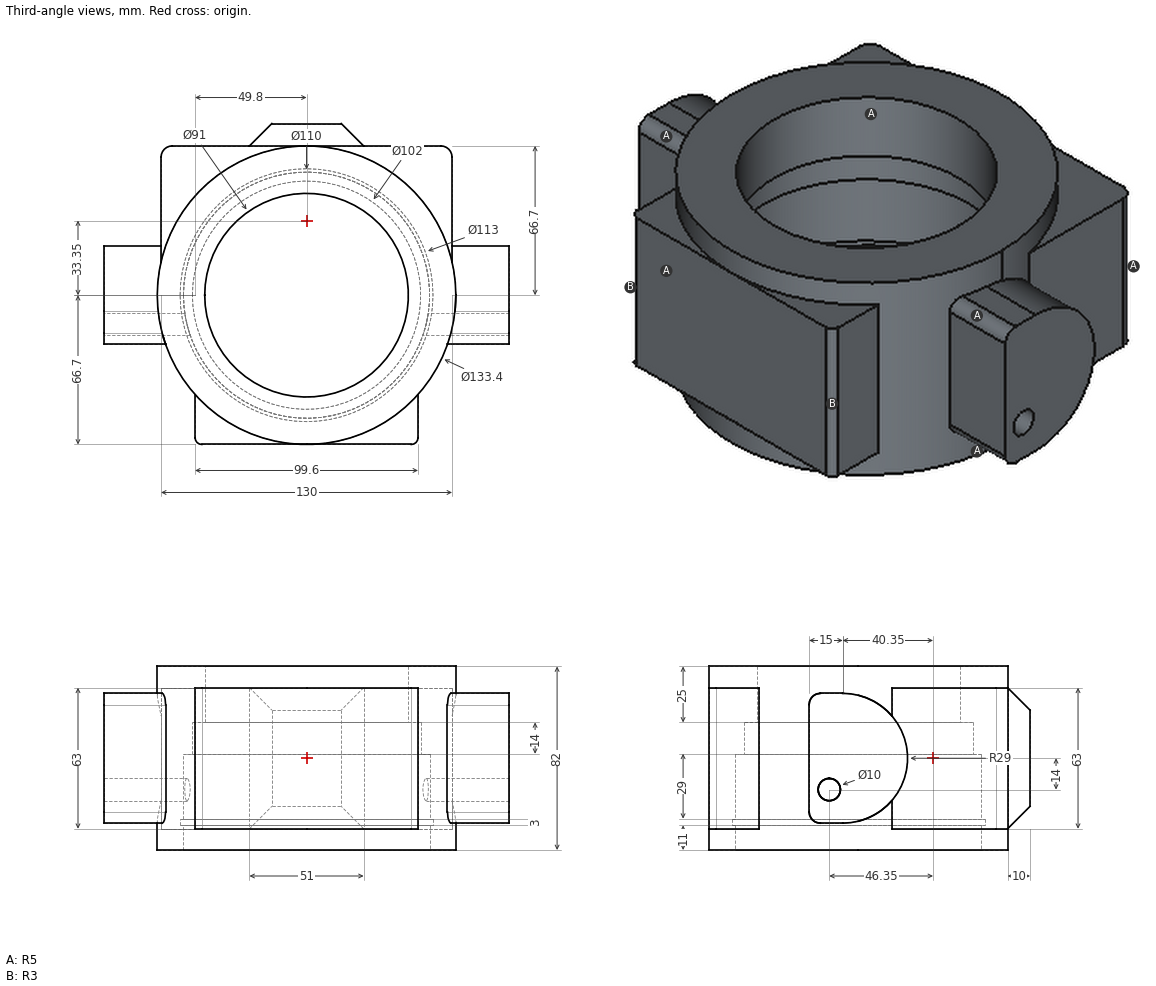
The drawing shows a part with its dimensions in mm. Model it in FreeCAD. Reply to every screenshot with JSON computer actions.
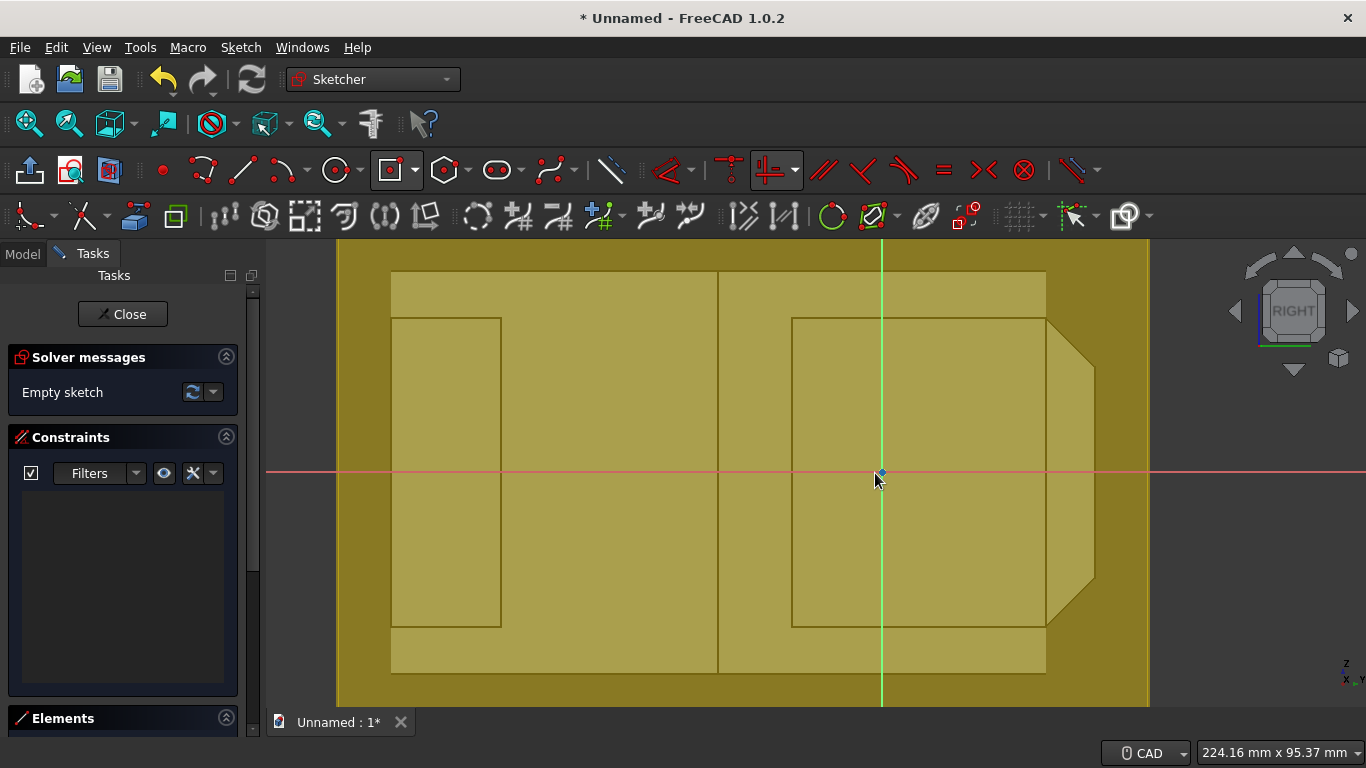
{"action": "key", "text": "g m"}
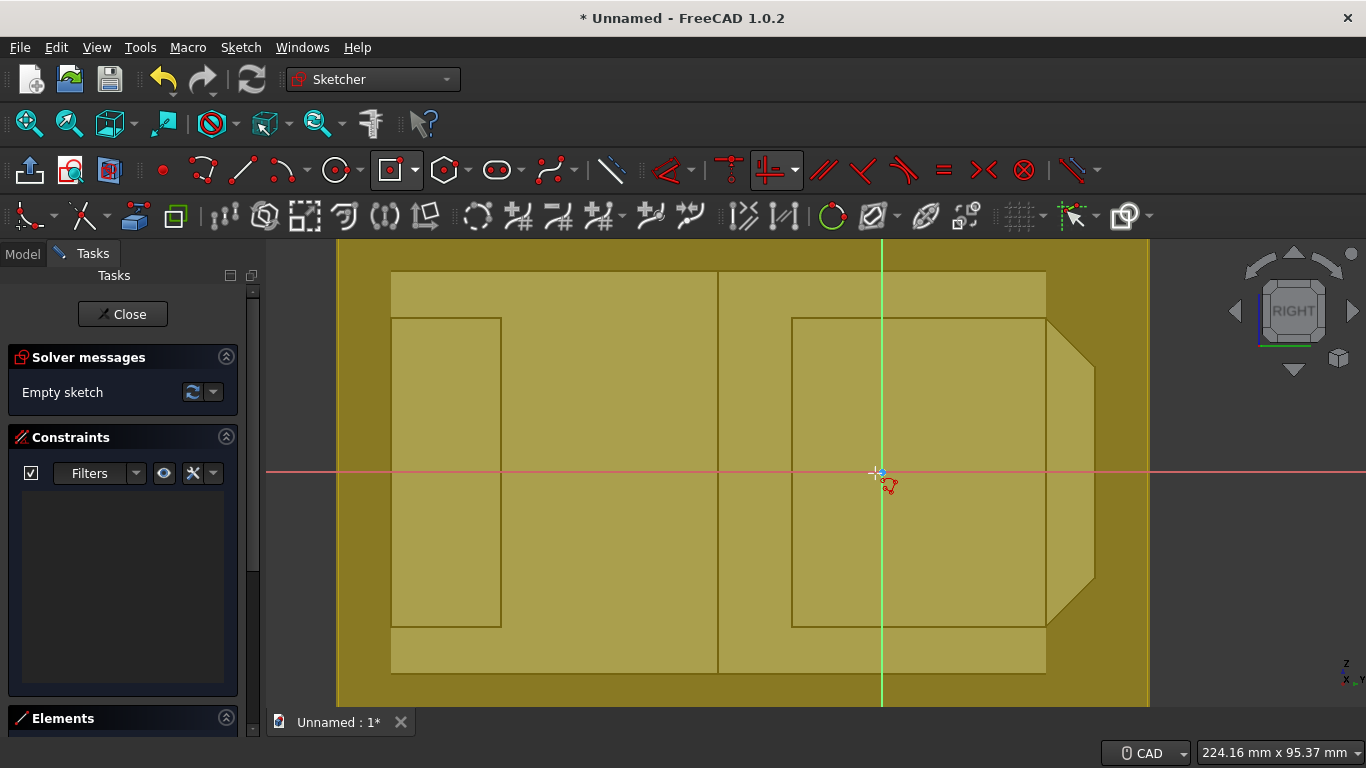
{"action": "left_click", "coordinate": [684, 330]}
{"action": "left_click", "coordinate": [611, 330]}
{"action": "left_click", "coordinate": [611, 615]}
{"action": "left_click", "coordinate": [684, 615]}
{"action": "right_click", "coordinate": [684, 615]}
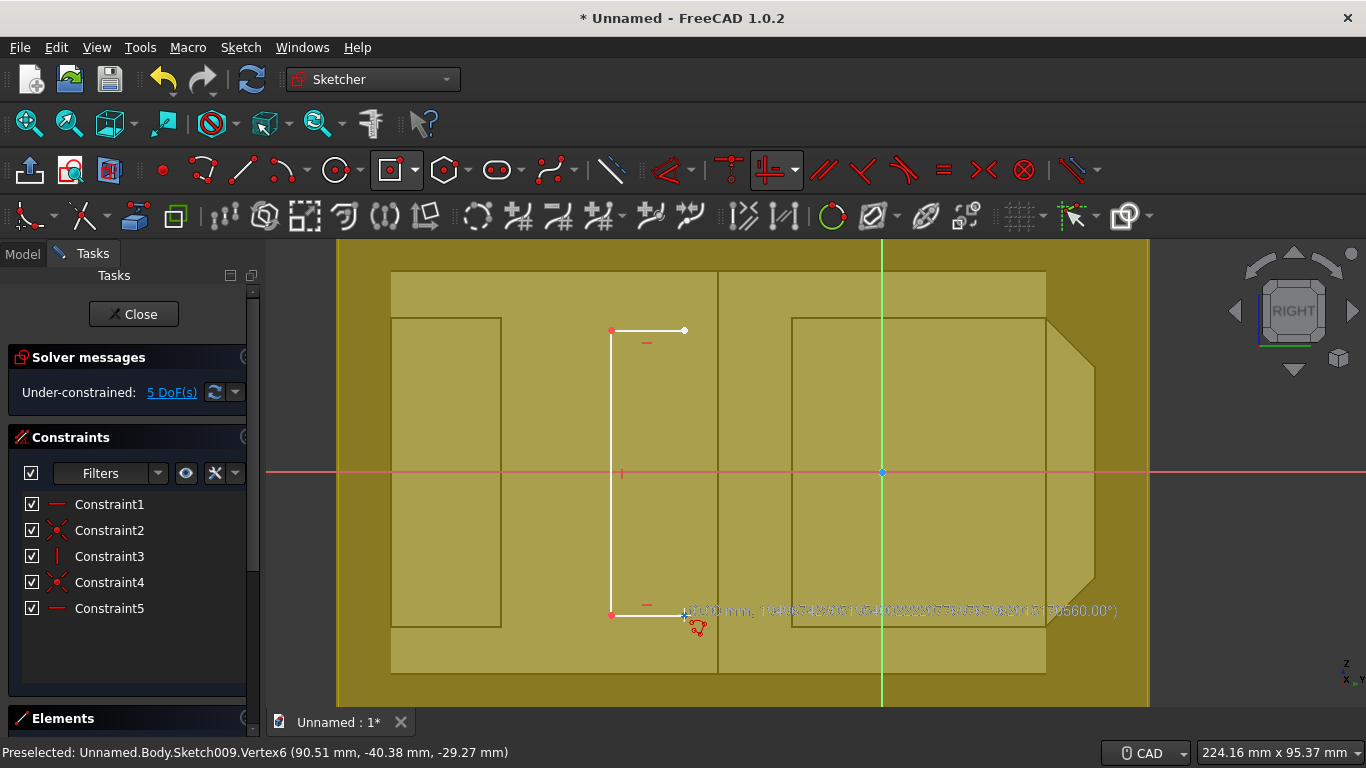
{"action": "key", "text": "g 3 a"}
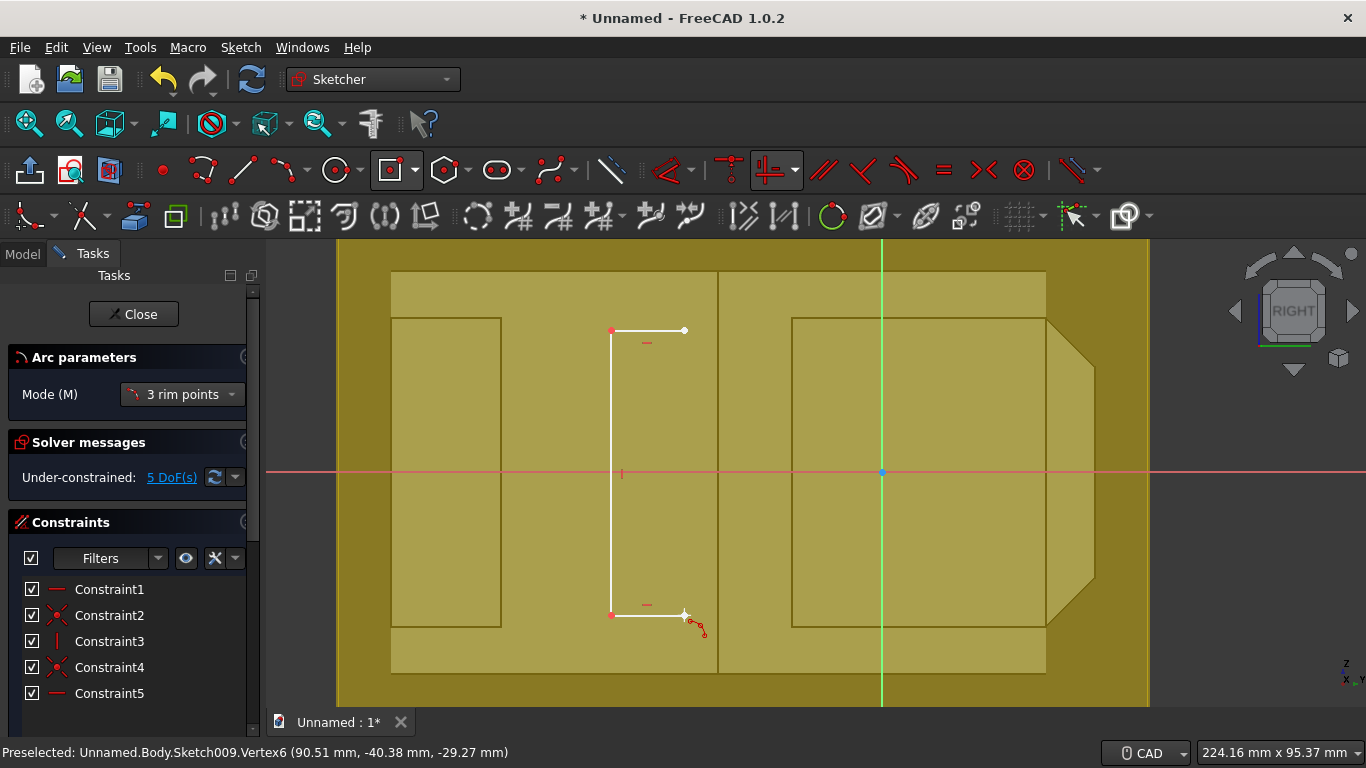
{"action": "left_click", "coordinate": [684, 616]}
{"action": "left_click", "coordinate": [684, 331]}
{"action": "left_click", "coordinate": [819, 516]}
{"action": "key", "text": "Escape"}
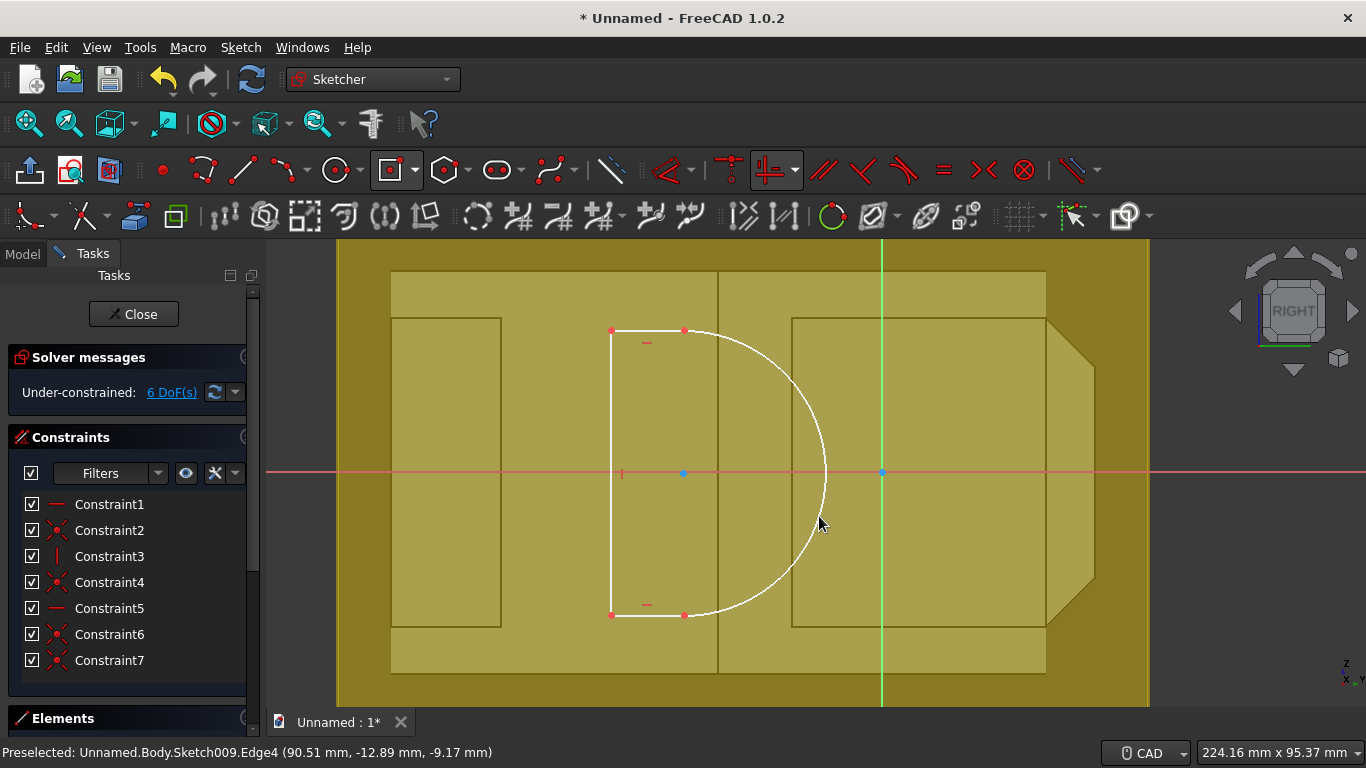
{"action": "left_click", "coordinate": [662, 331]}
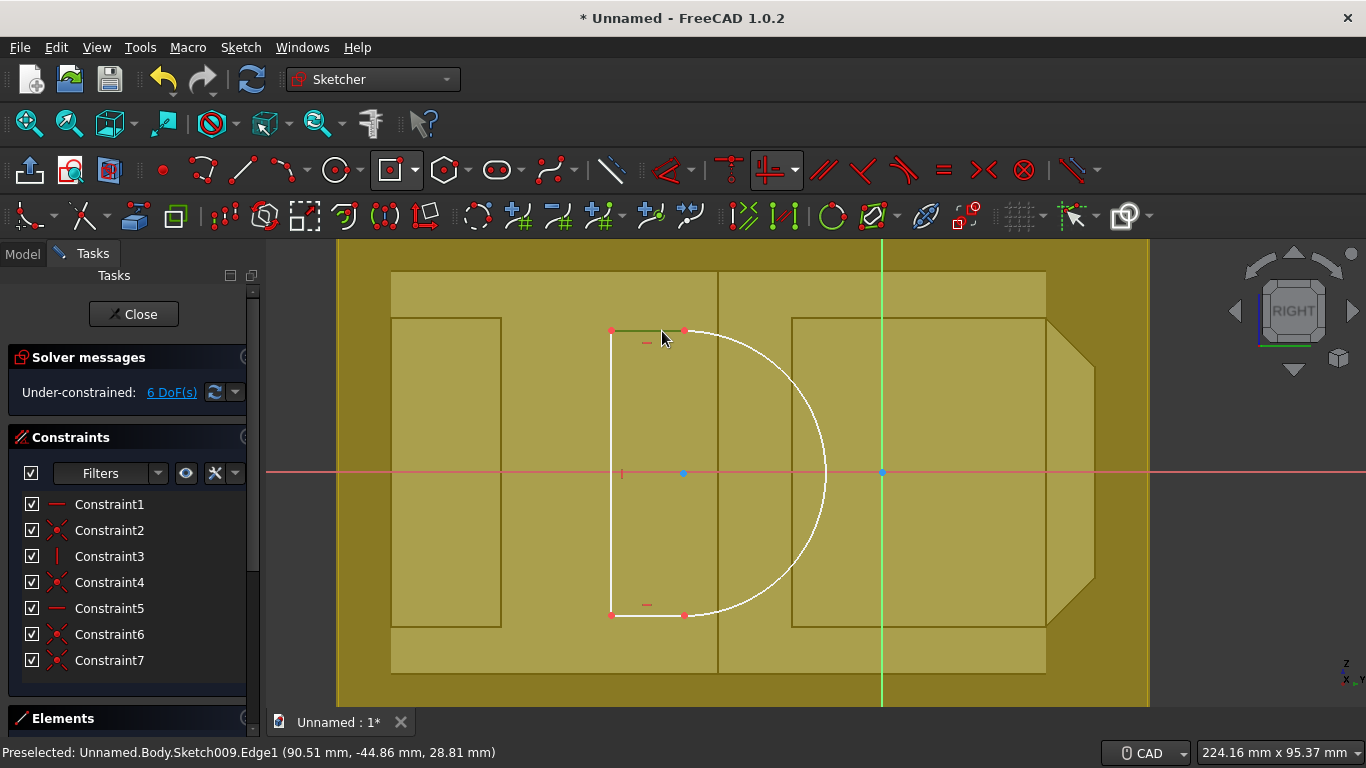
{"action": "left_click", "coordinate": [799, 557]}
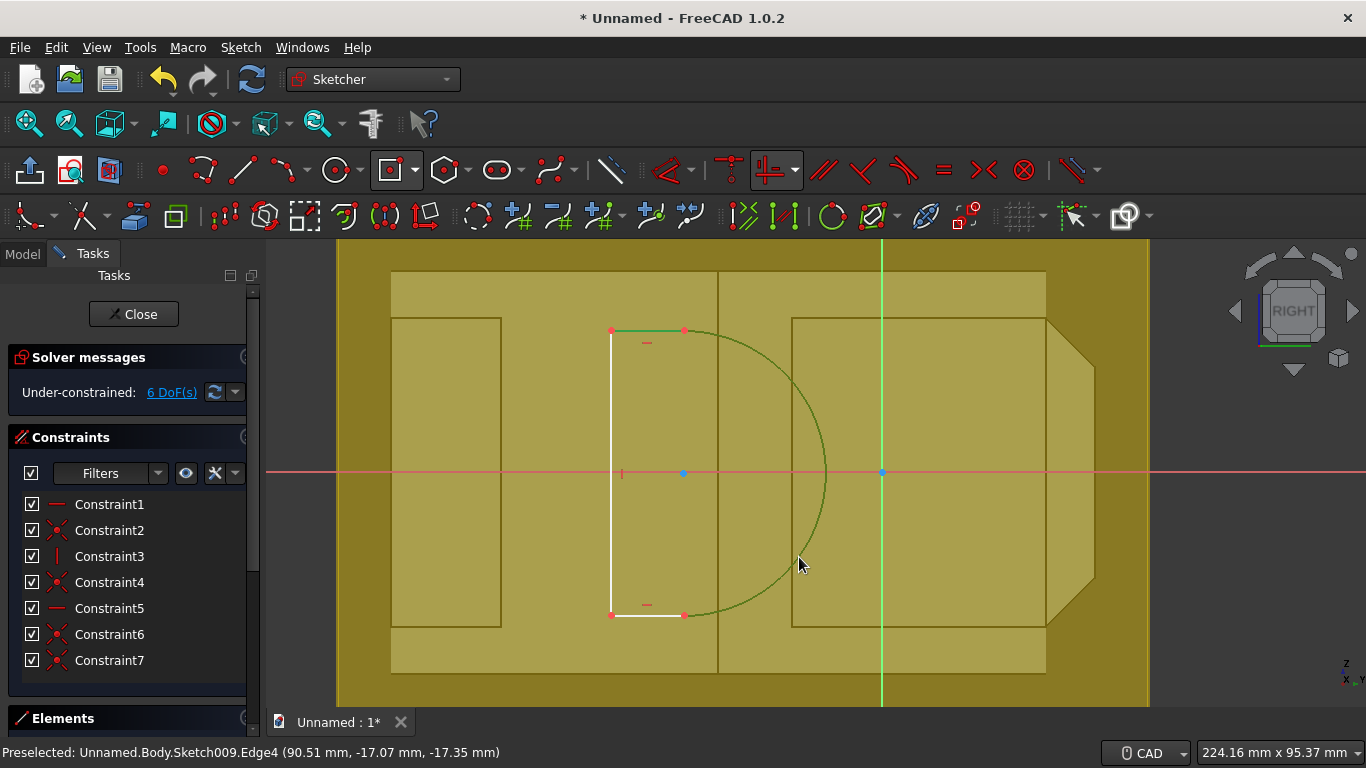
{"action": "key", "text": "t"}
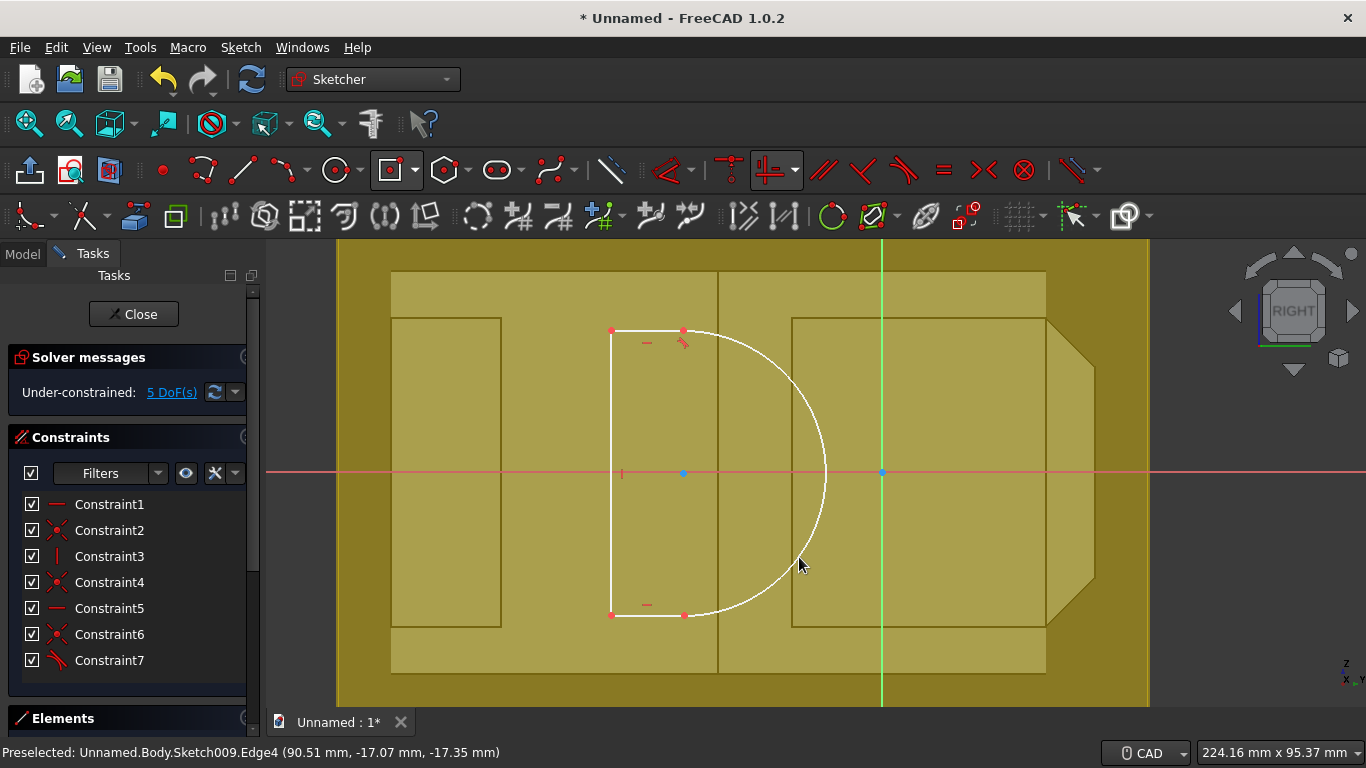
{"action": "left_click", "coordinate": [633, 616]}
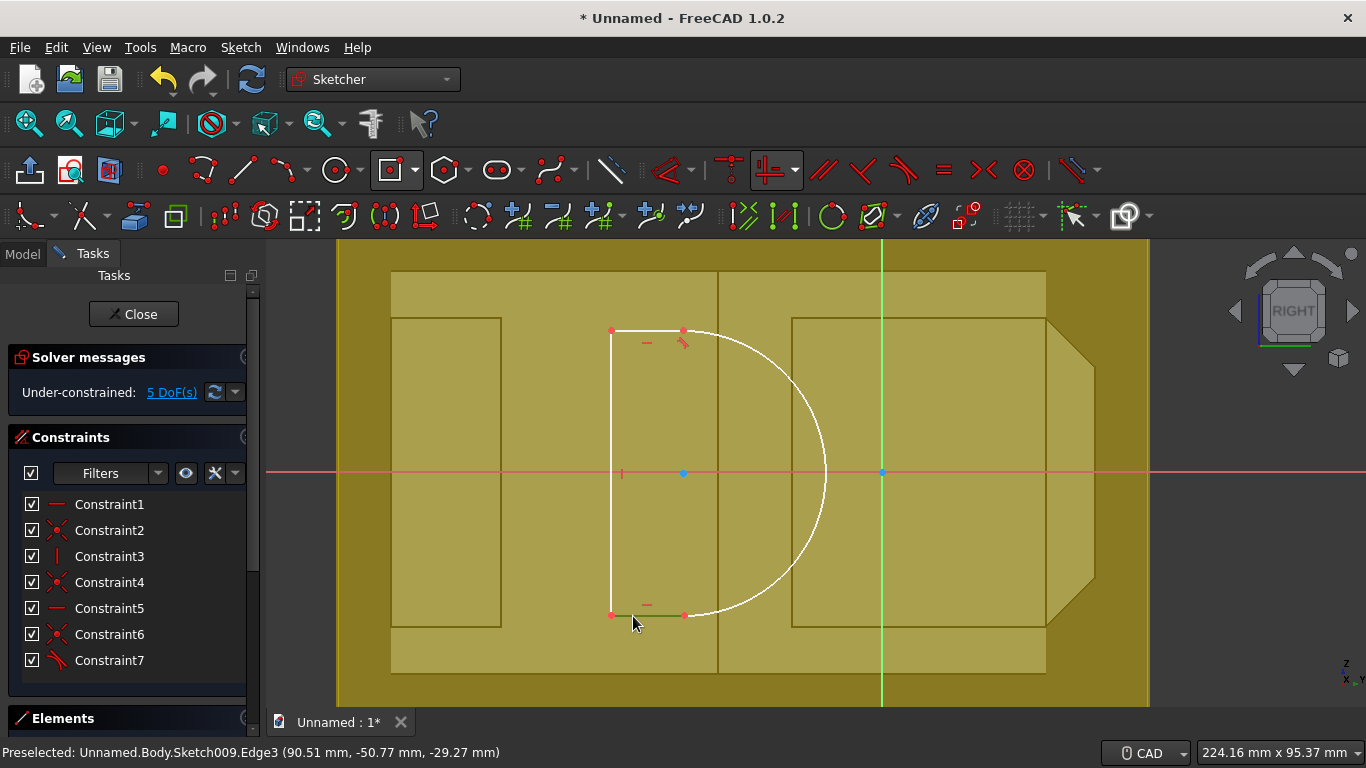
{"action": "left_click", "coordinate": [799, 557]}